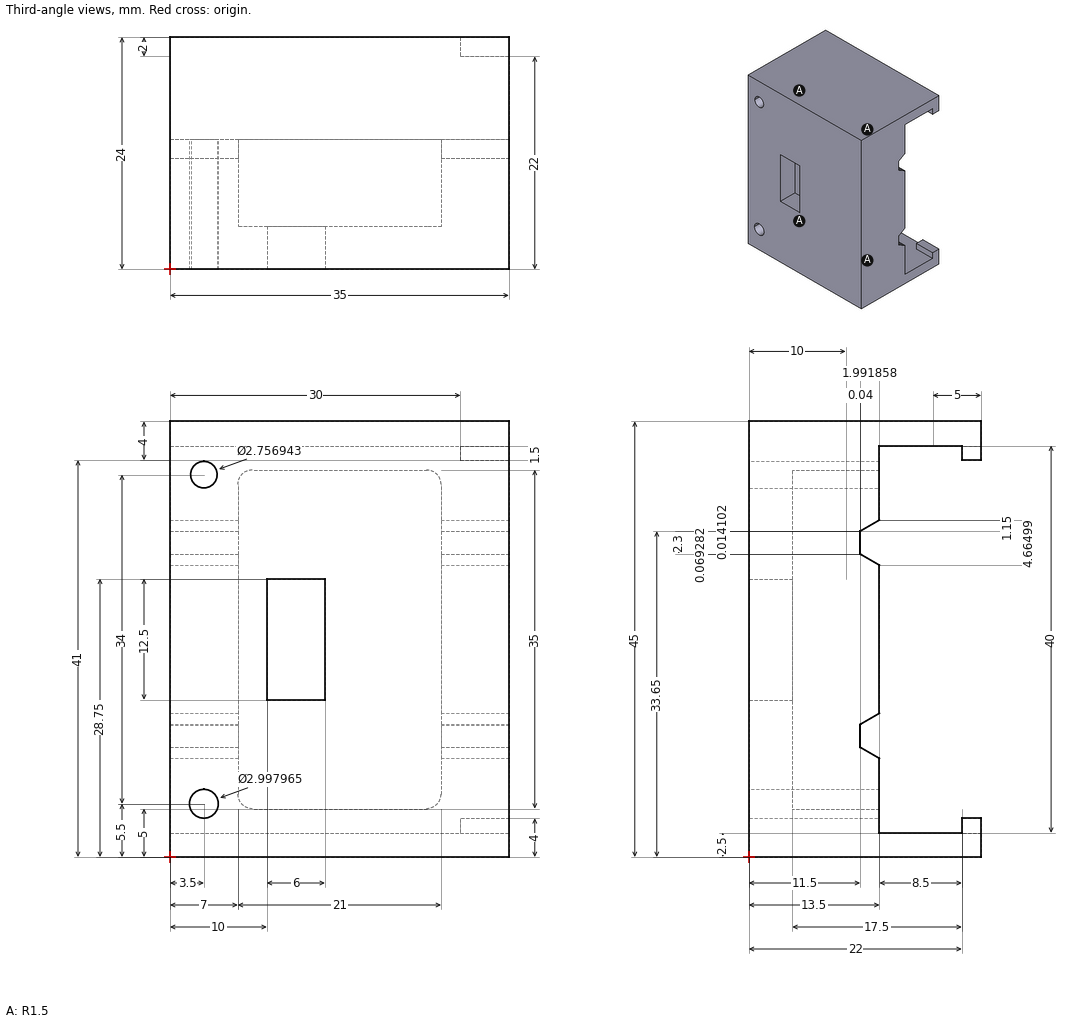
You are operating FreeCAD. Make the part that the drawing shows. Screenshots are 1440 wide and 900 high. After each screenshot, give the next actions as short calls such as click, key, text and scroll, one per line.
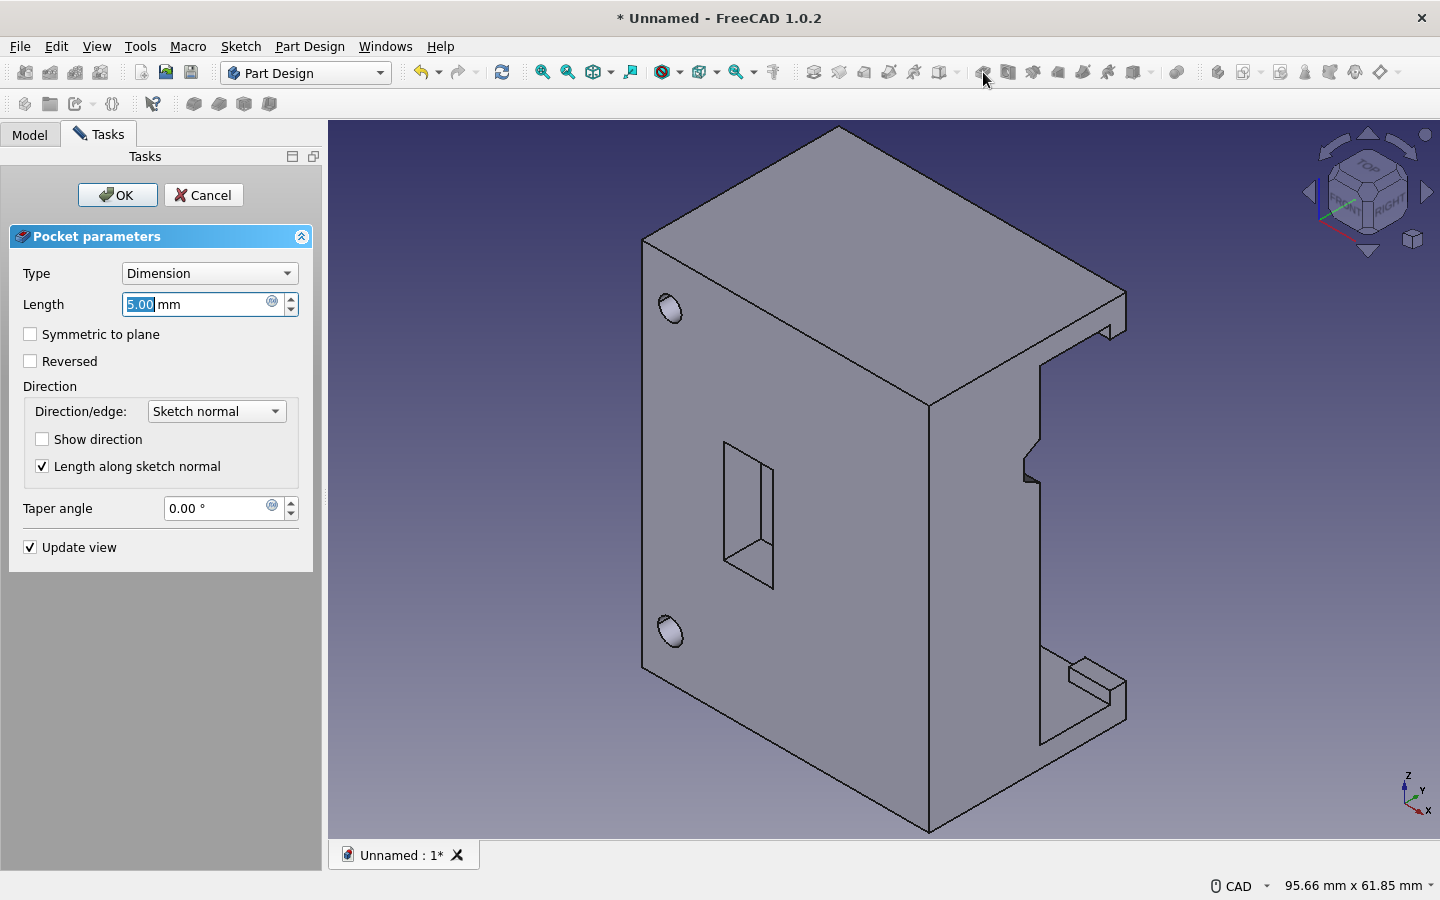
click(210, 274)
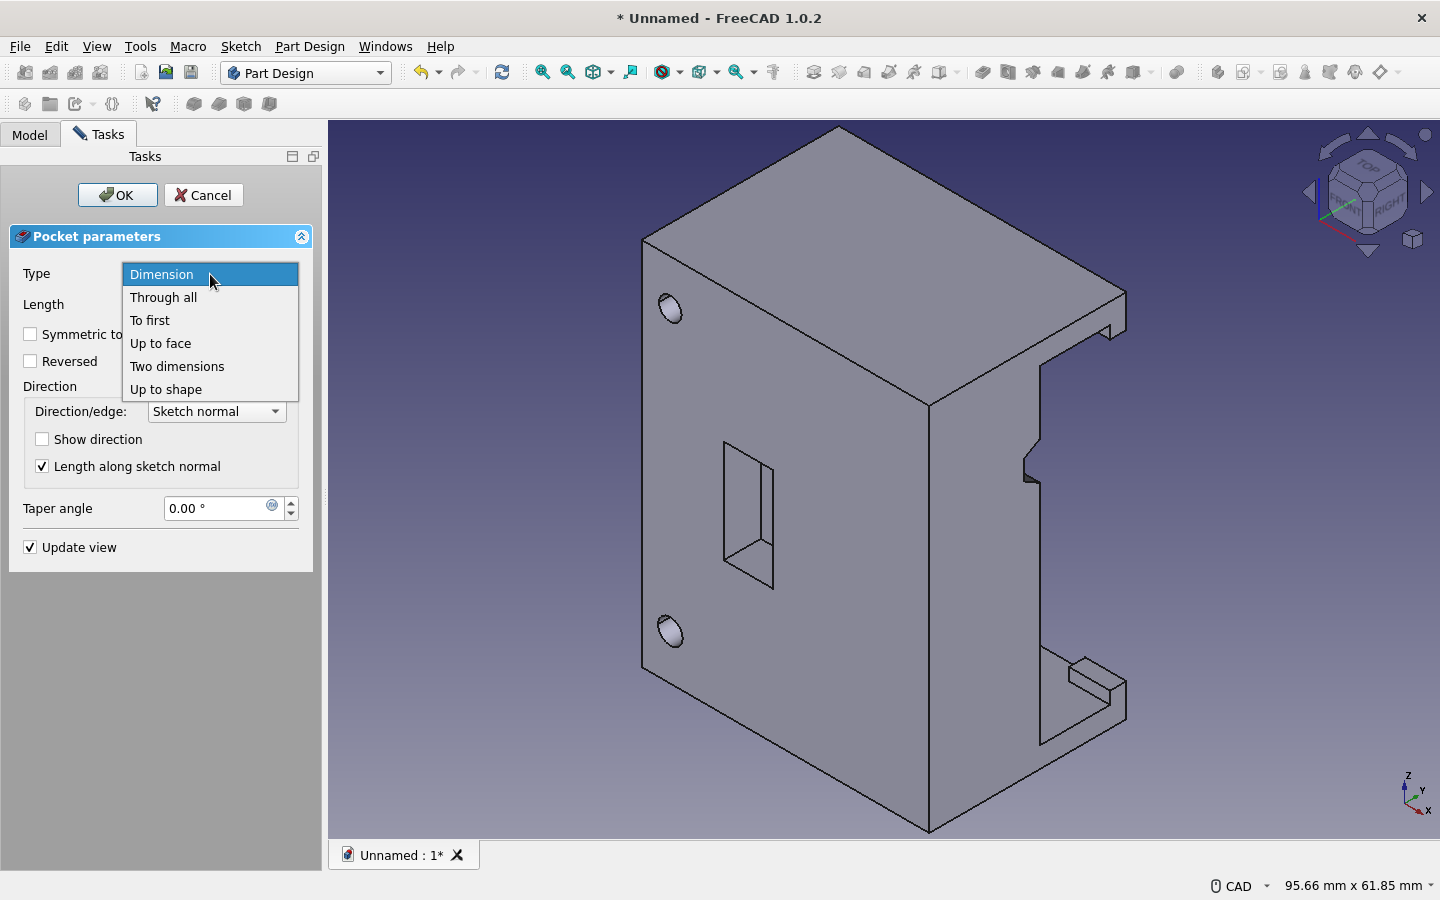
click(208, 298)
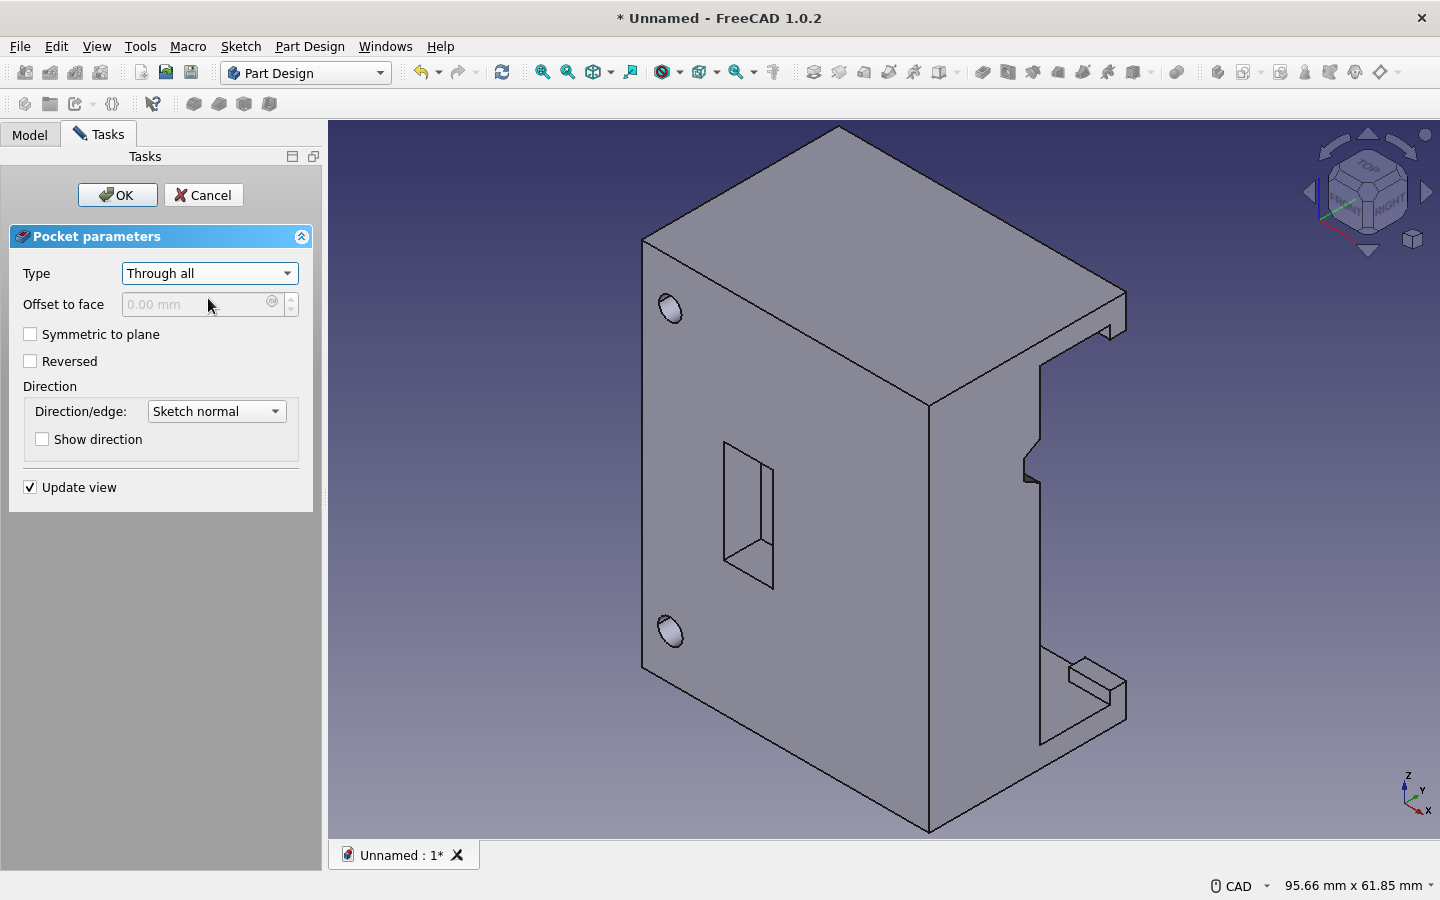
click(118, 195)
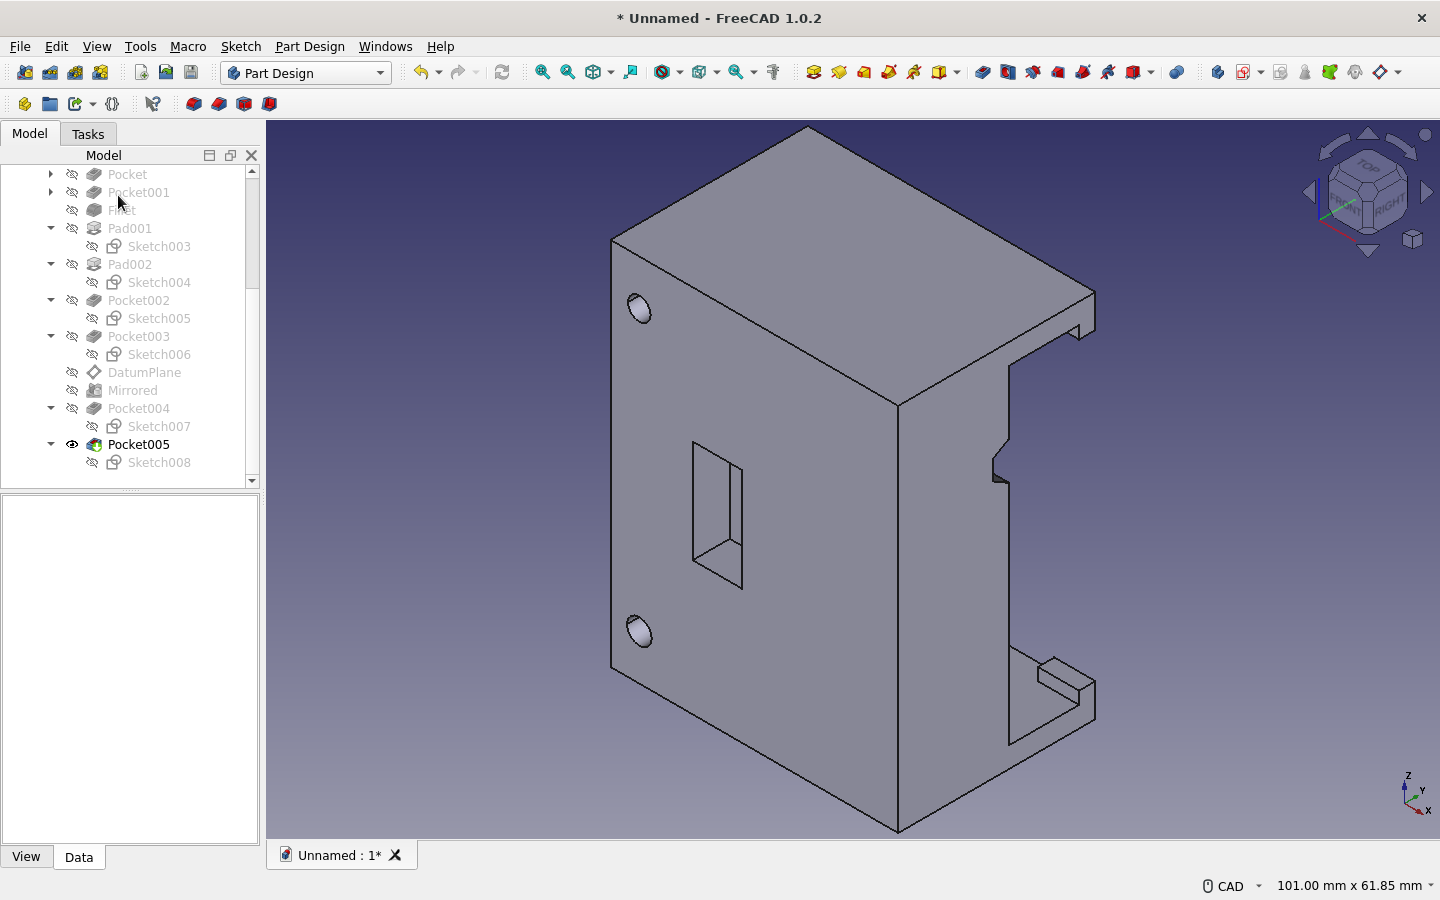
scroll(141, 314, down, 3)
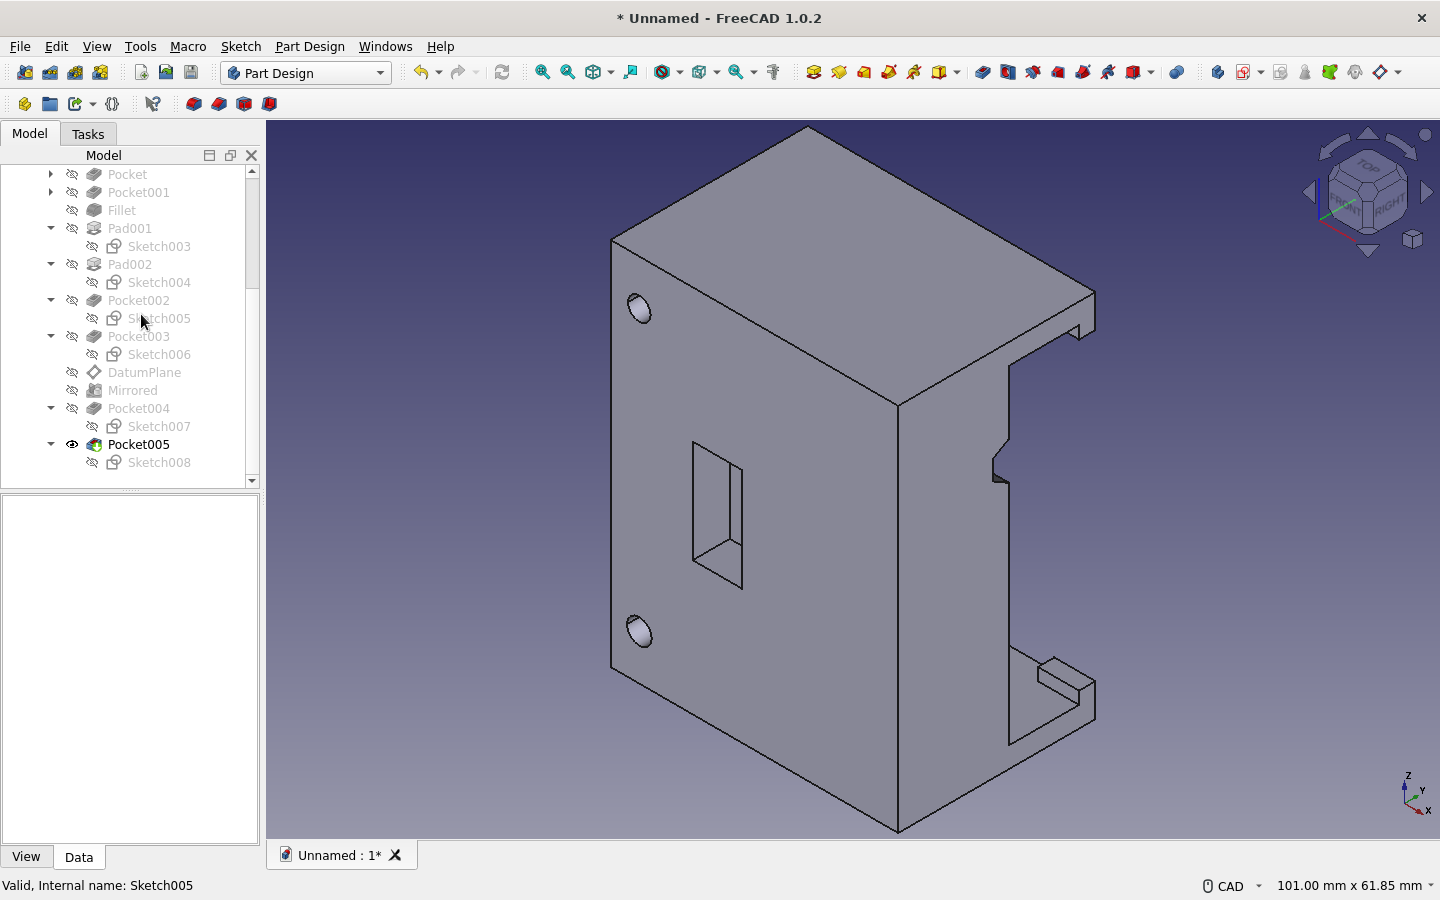
scroll(141, 314, up, 15)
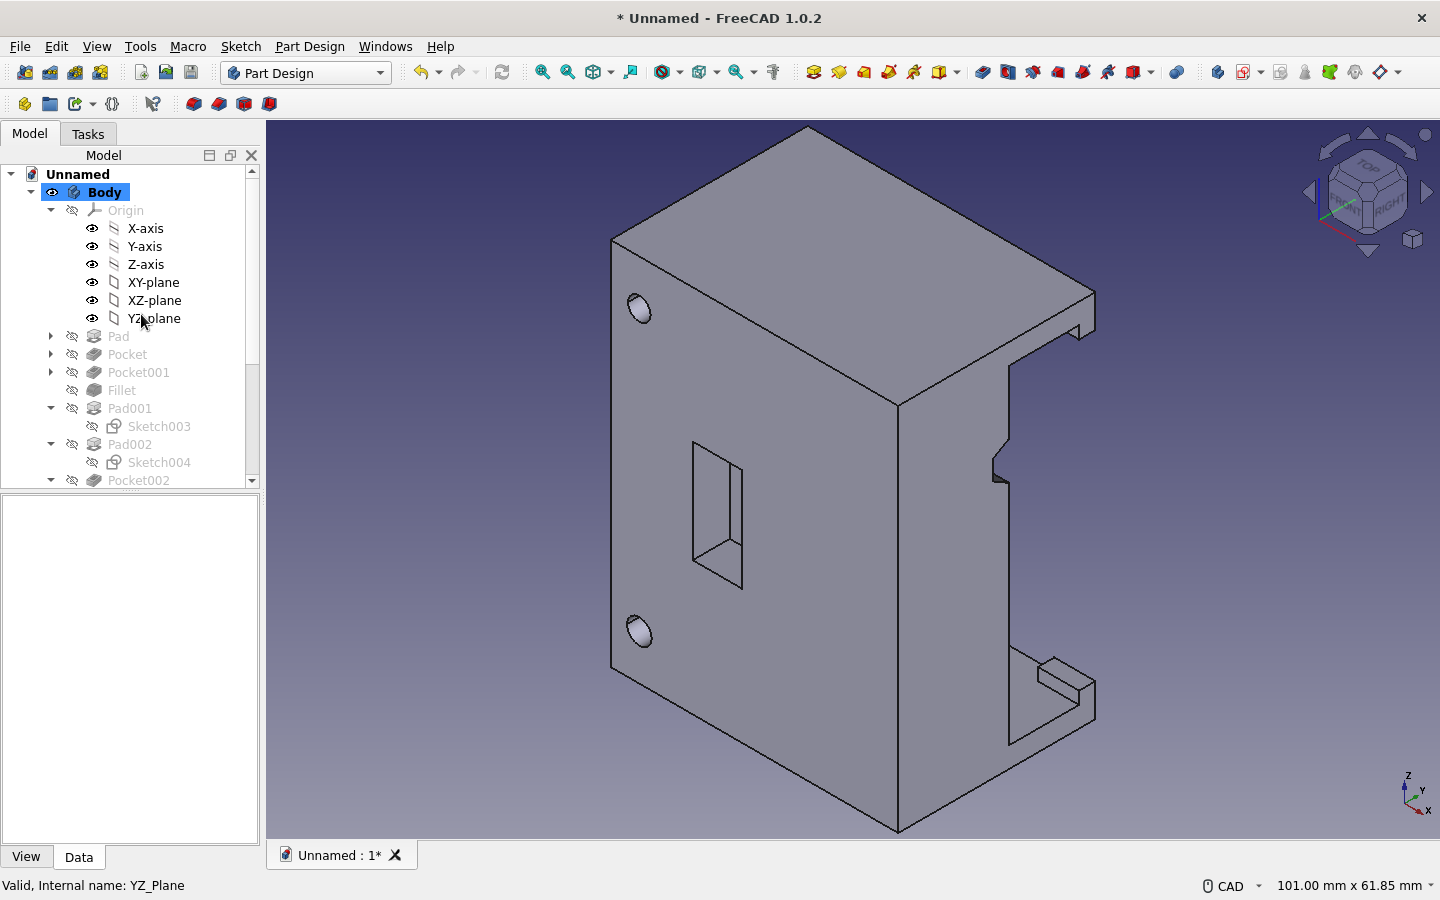
click(137, 282)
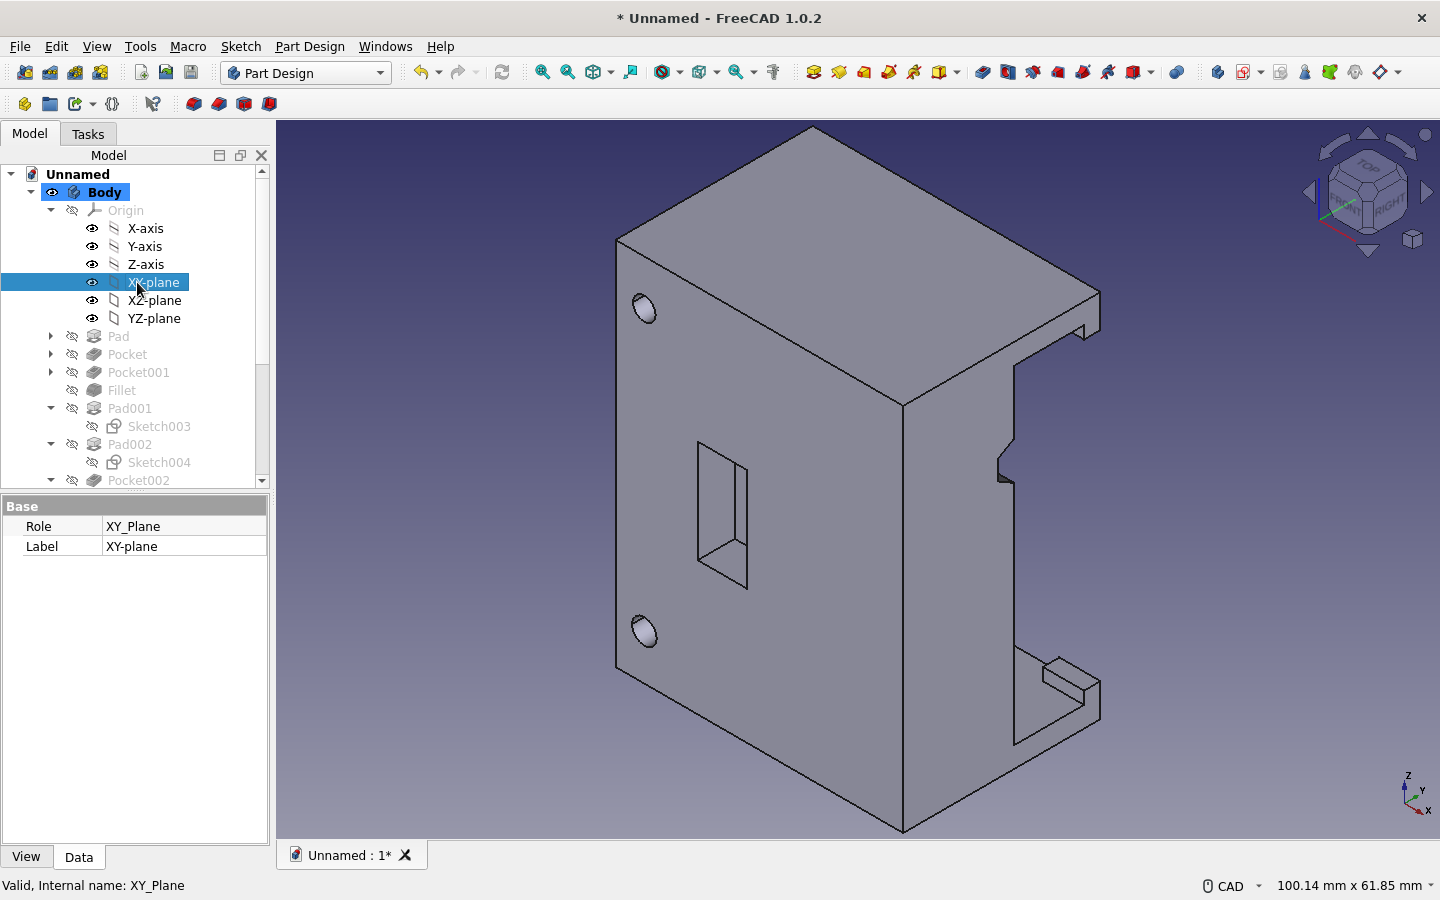
click(1380, 72)